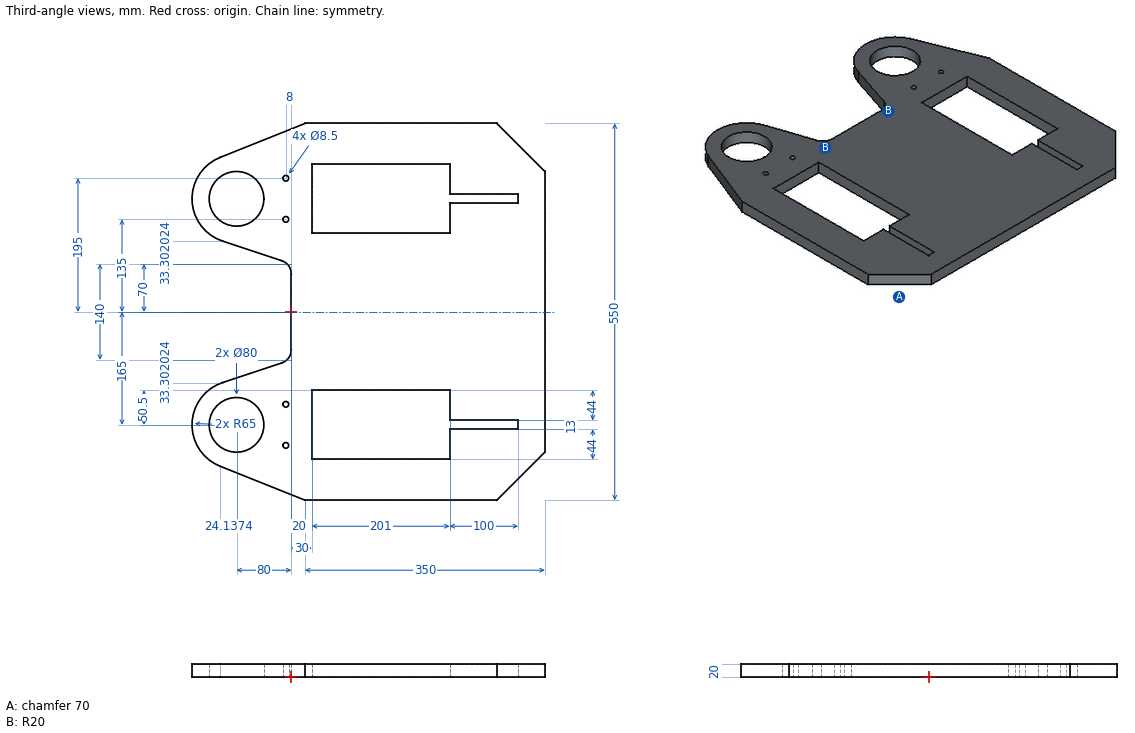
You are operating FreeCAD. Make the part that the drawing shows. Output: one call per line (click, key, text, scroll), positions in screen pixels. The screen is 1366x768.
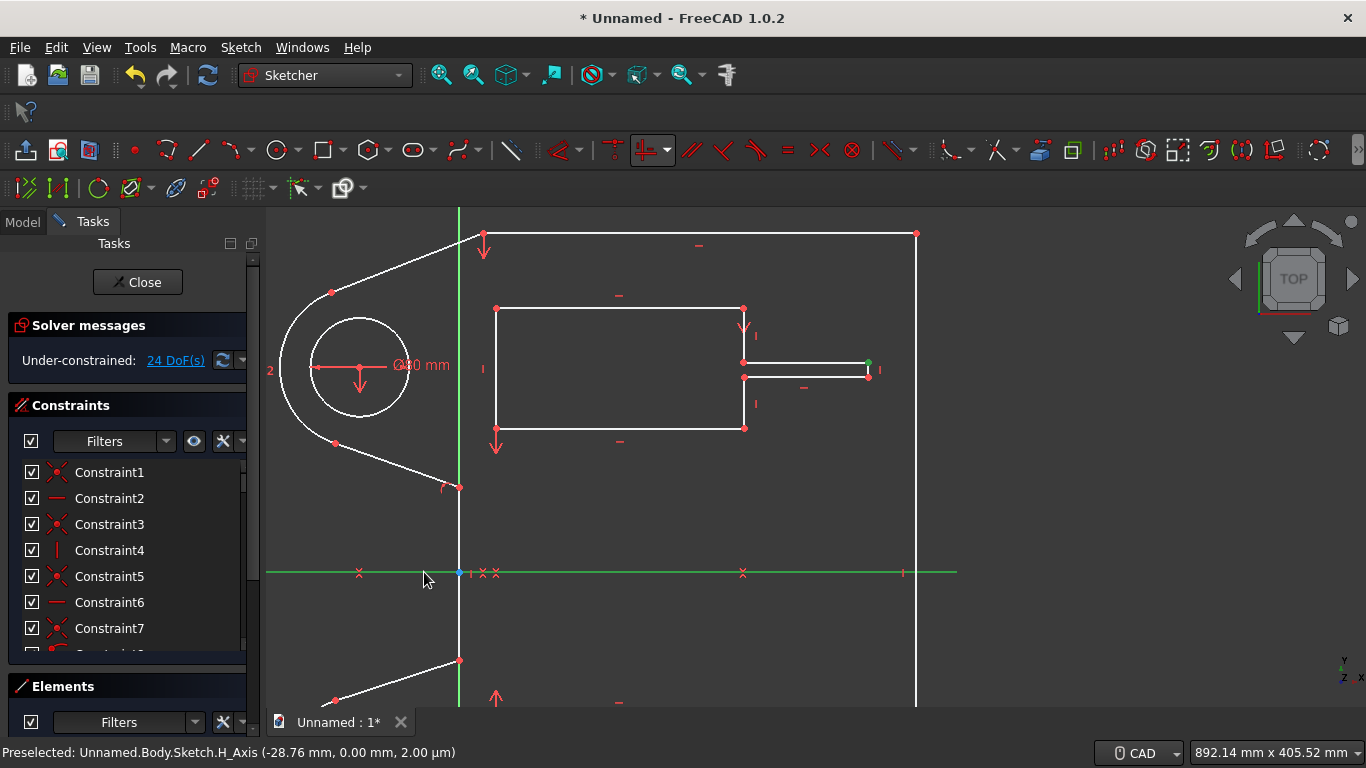
key(s)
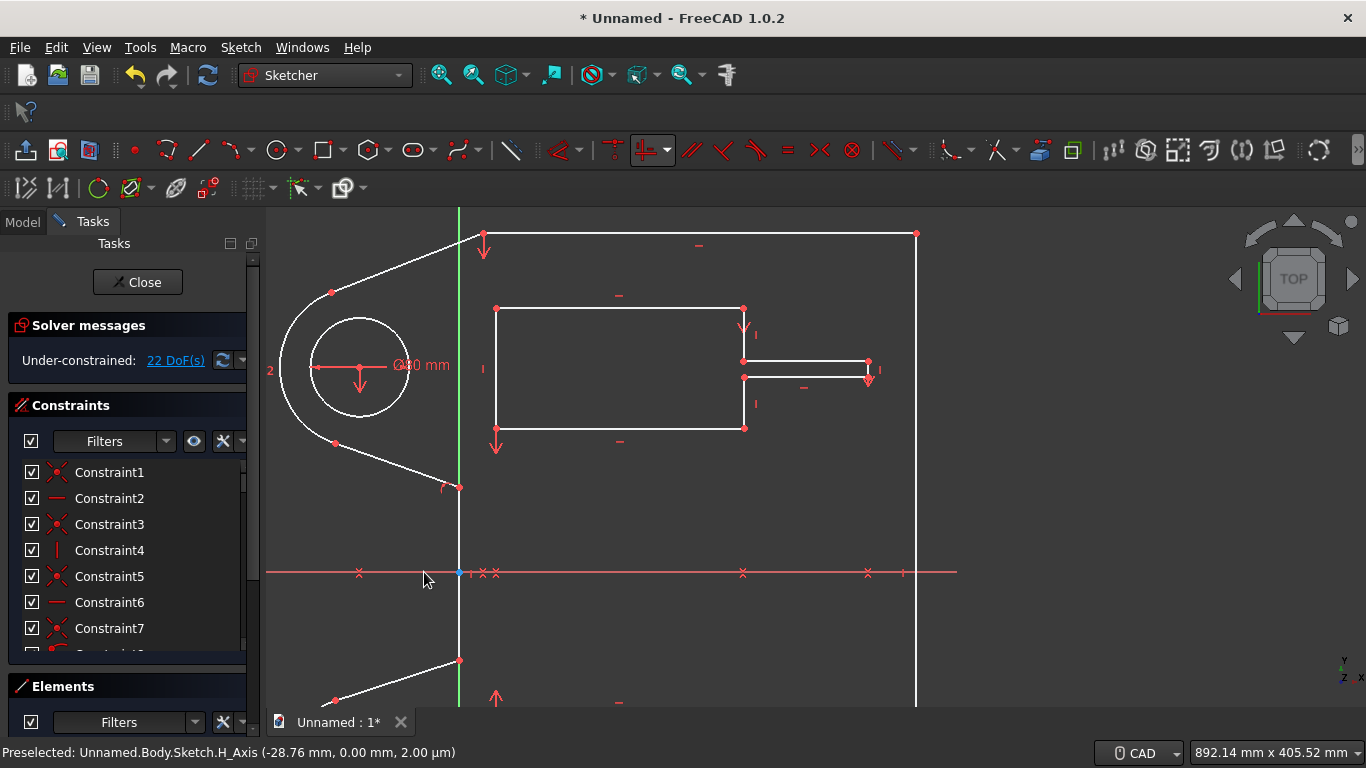
scroll(869, 363, down, 4)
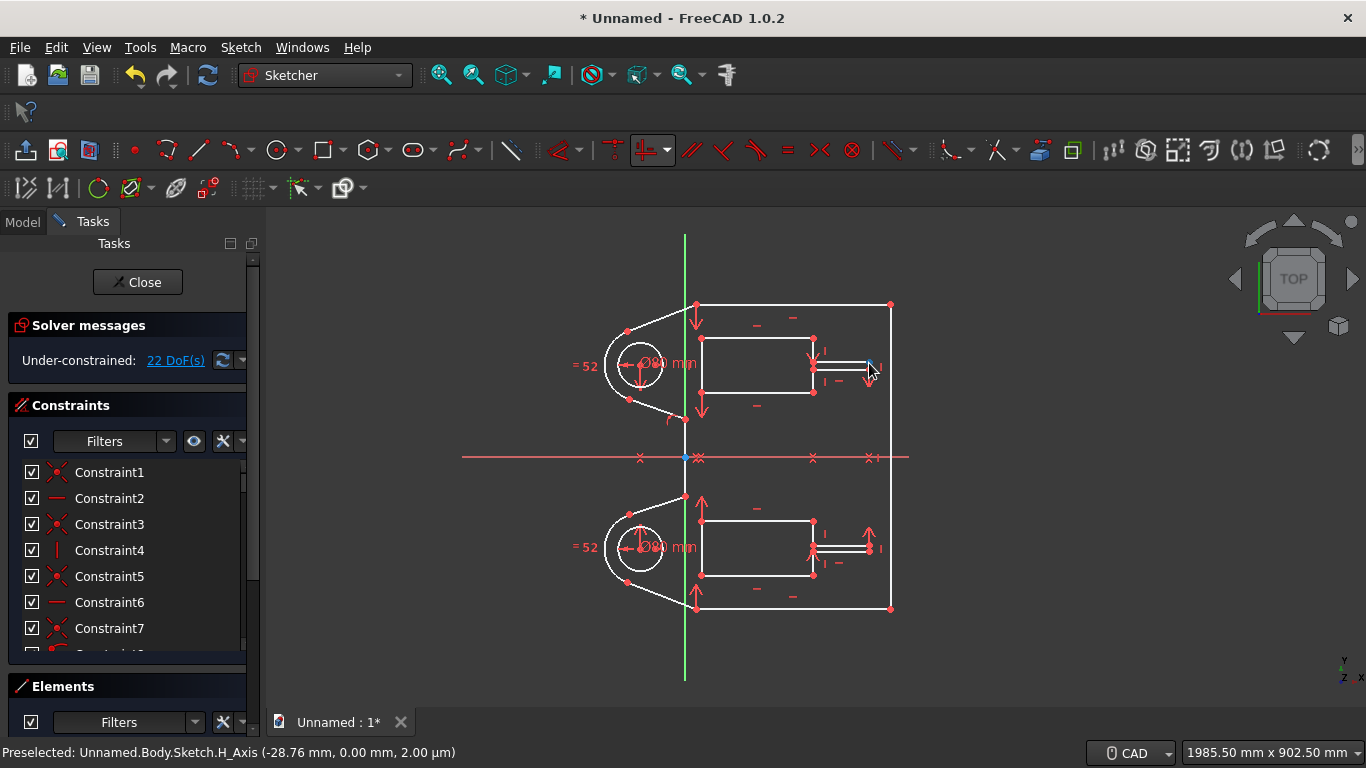
scroll(813, 546, up, 4)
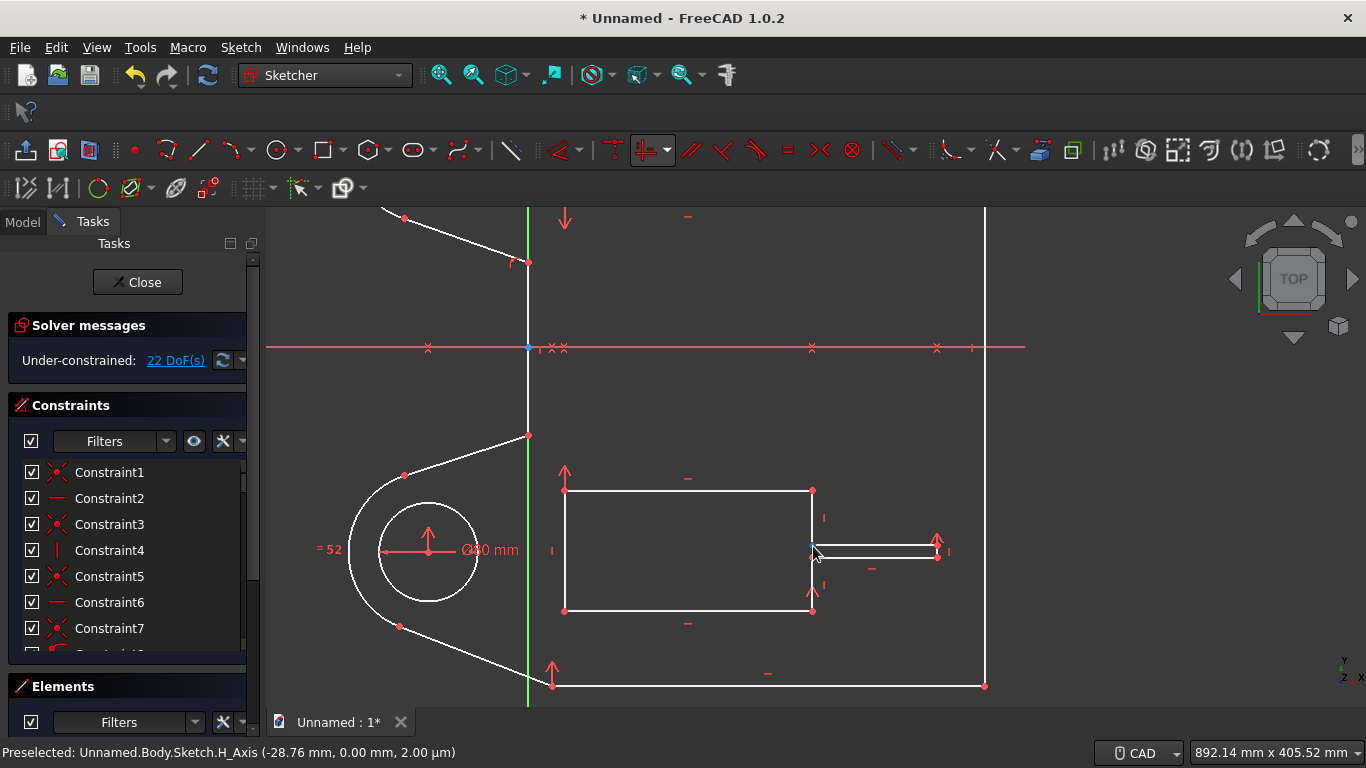
click(812, 545)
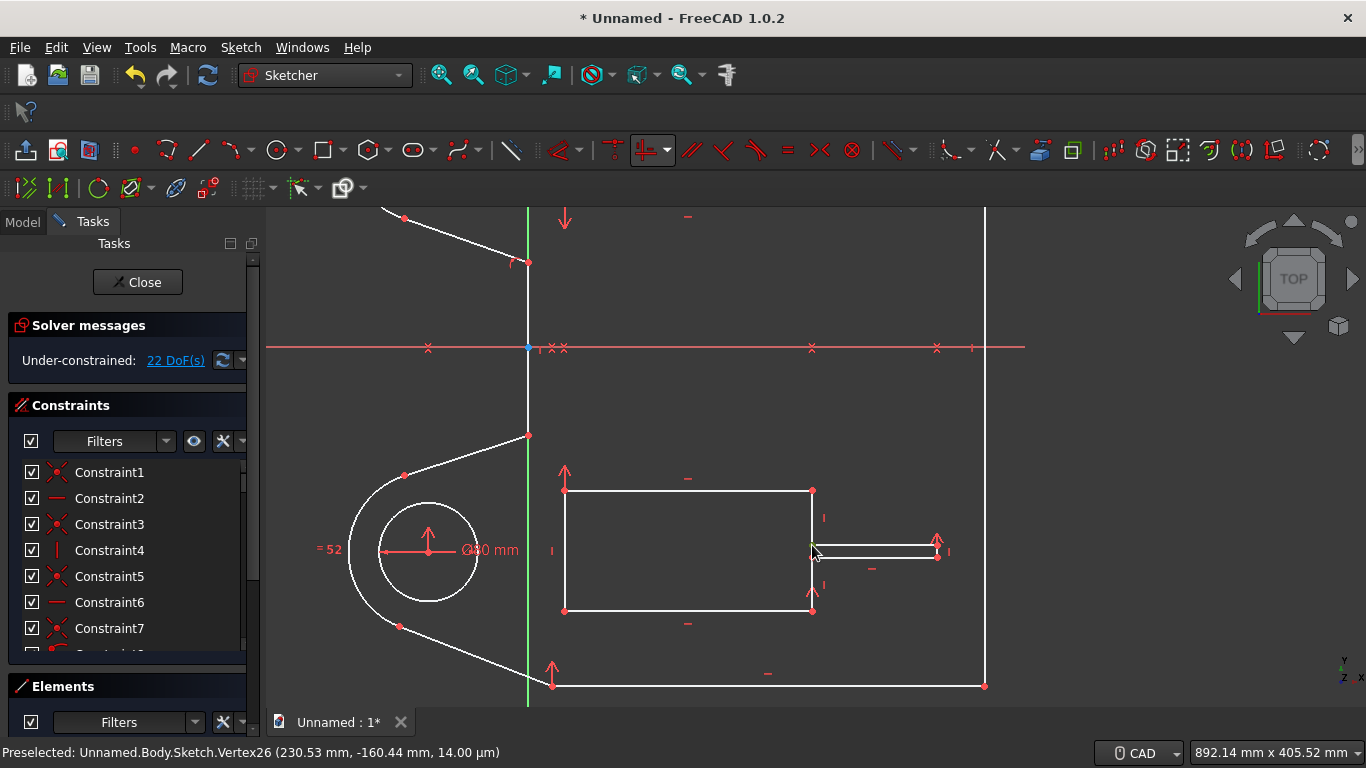
scroll(813, 546, down, 4)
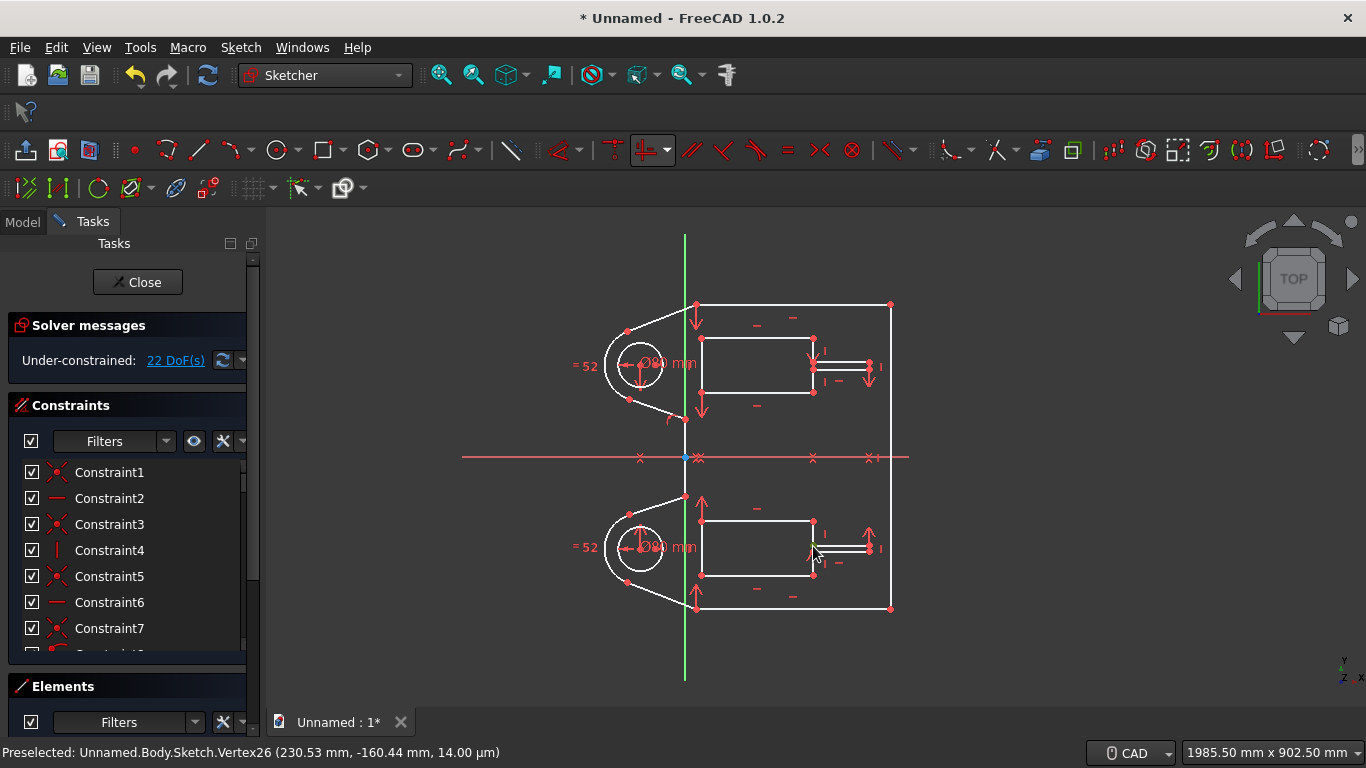
scroll(813, 370, up, 3)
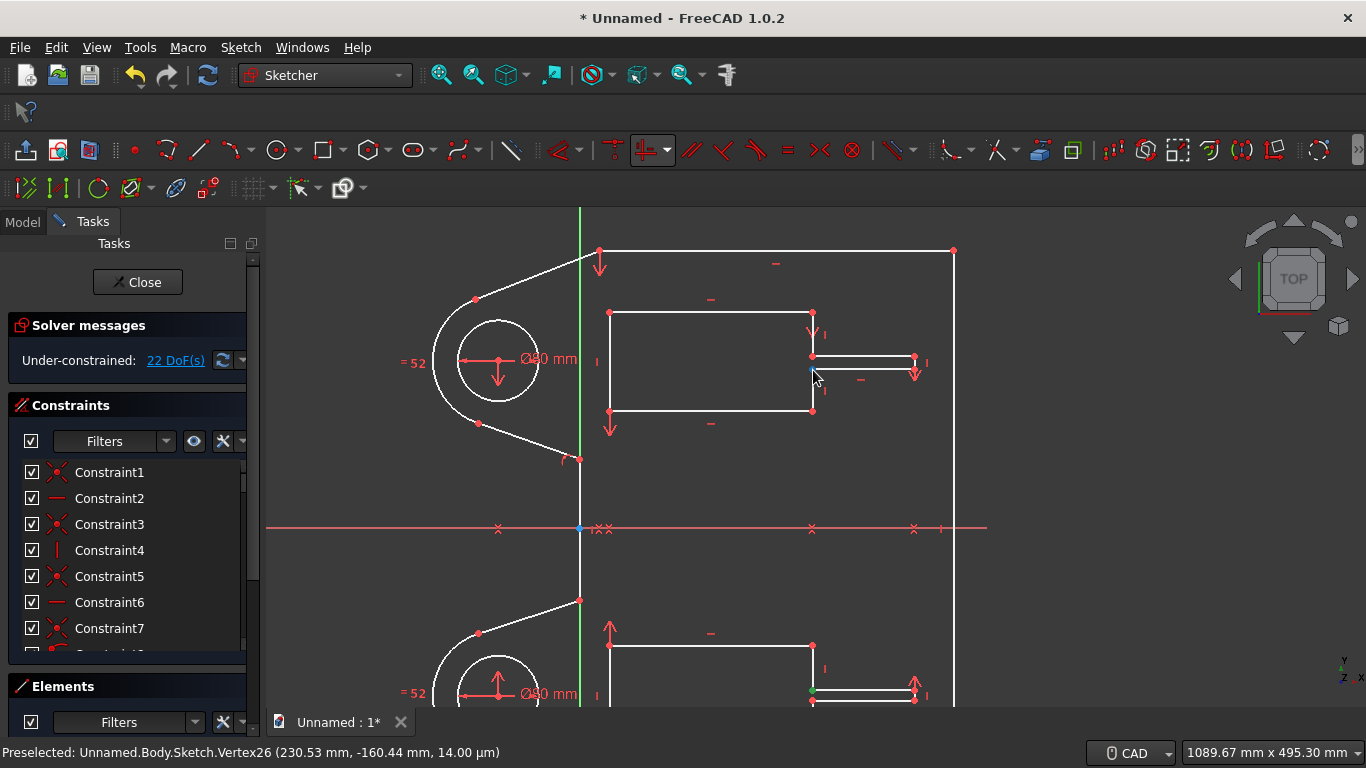
click(813, 369)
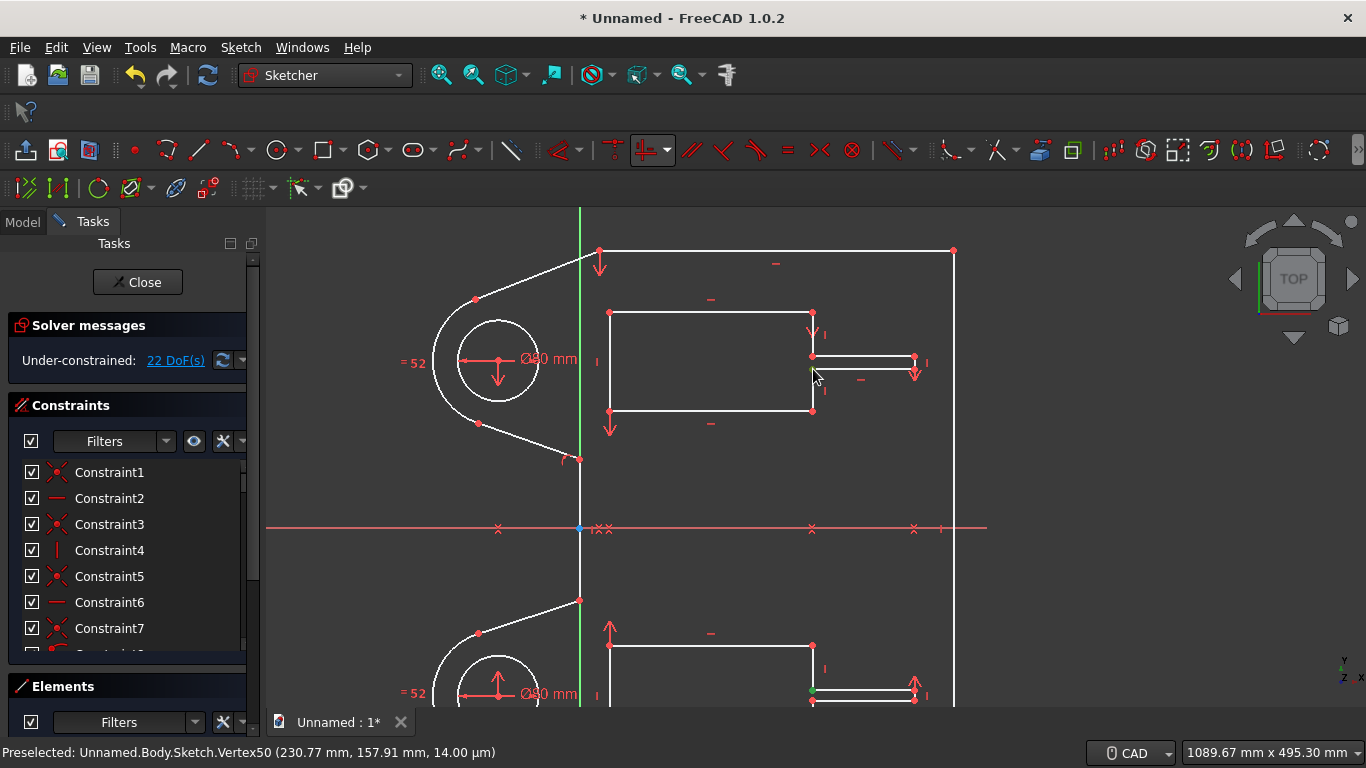
click(359, 528)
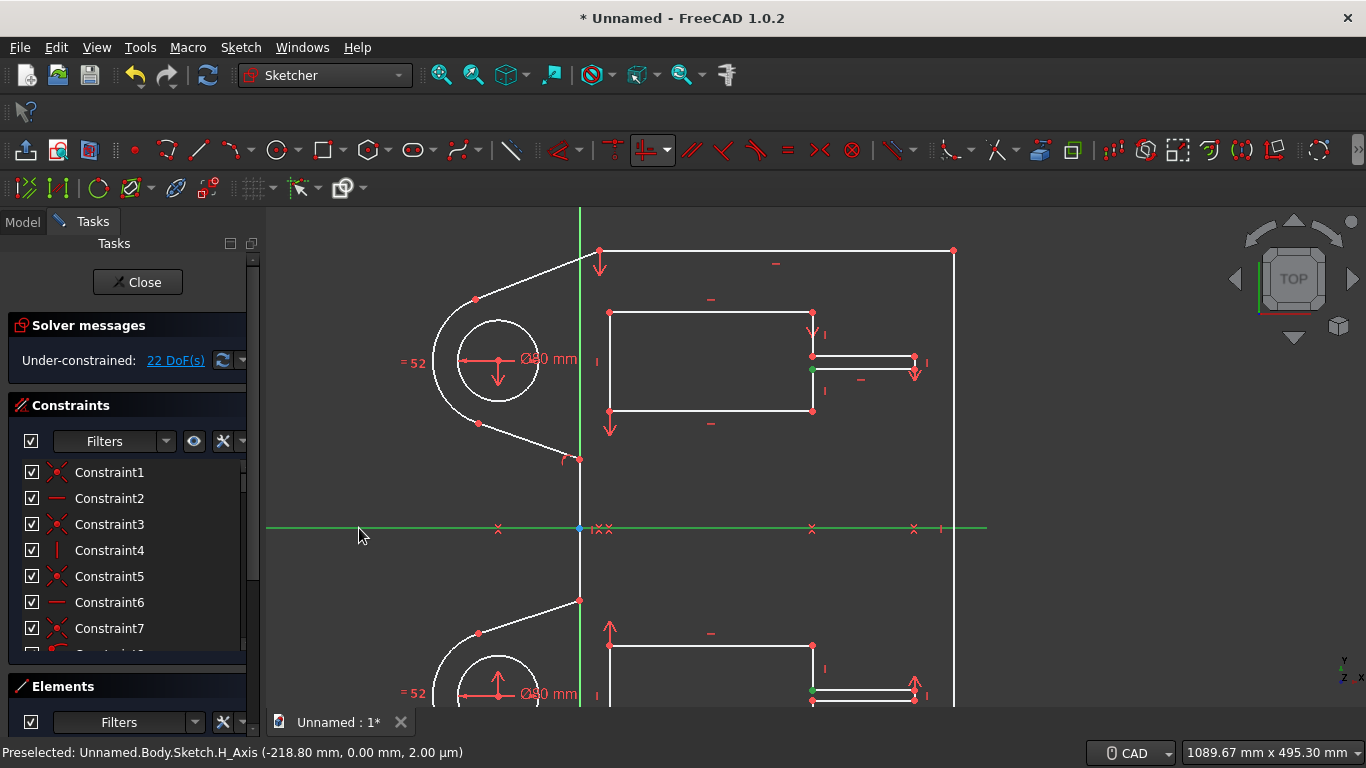
click(820, 150)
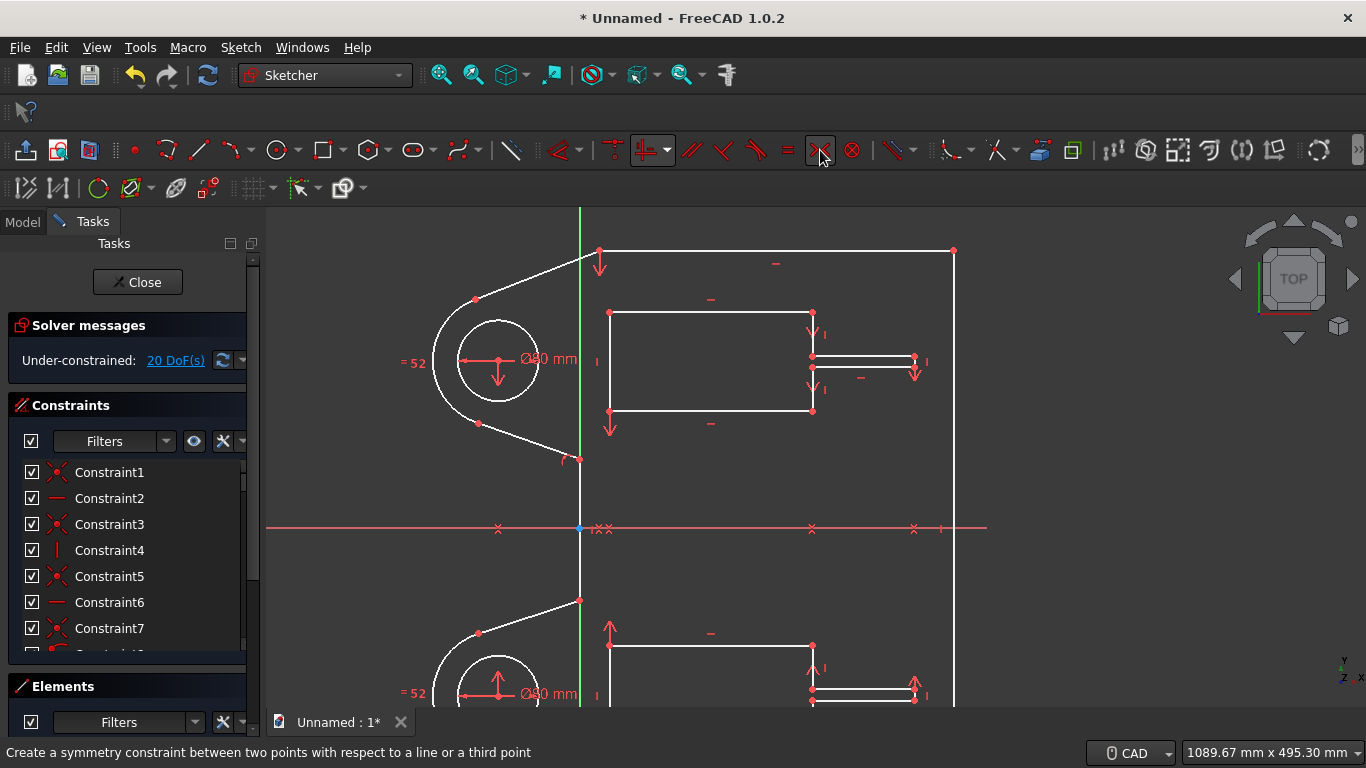
click(440, 331)